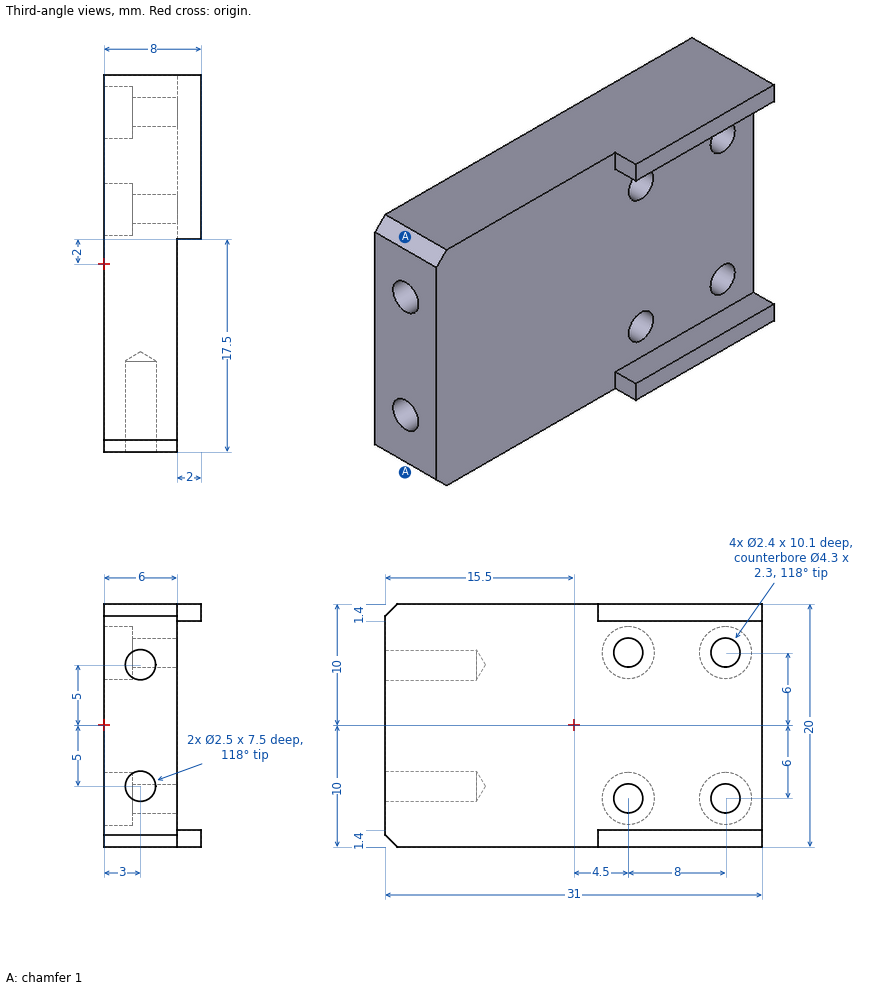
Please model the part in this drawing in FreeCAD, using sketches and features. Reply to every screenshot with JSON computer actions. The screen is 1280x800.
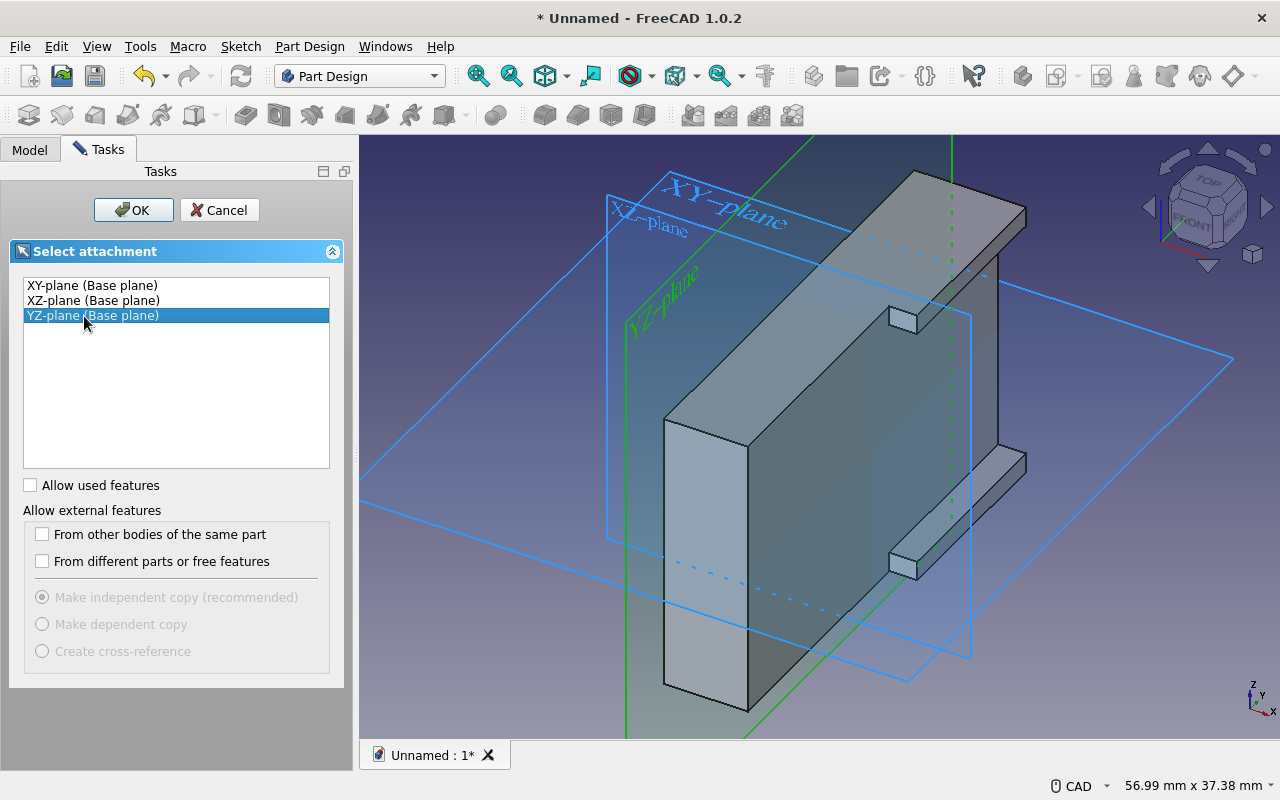
{"action": "left_click", "coordinate": [134, 210]}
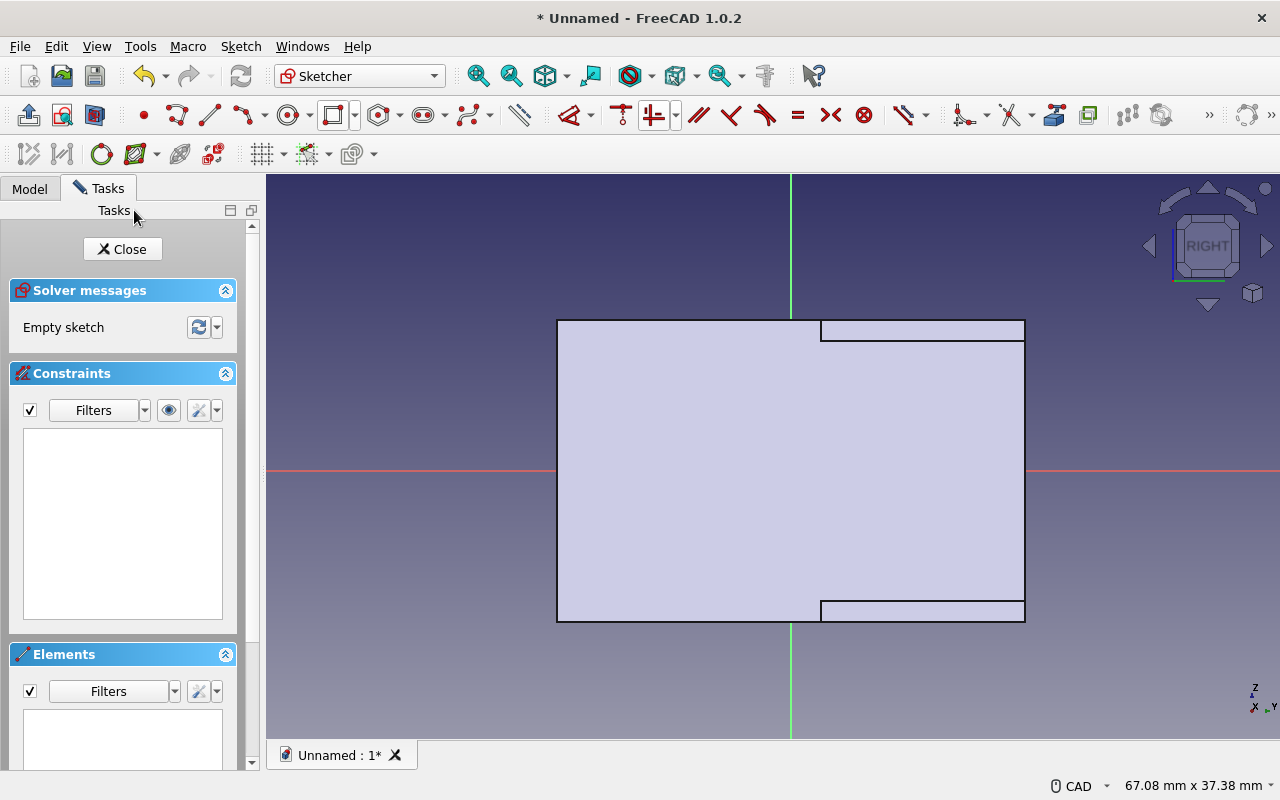
{"action": "left_click", "coordinate": [95, 116]}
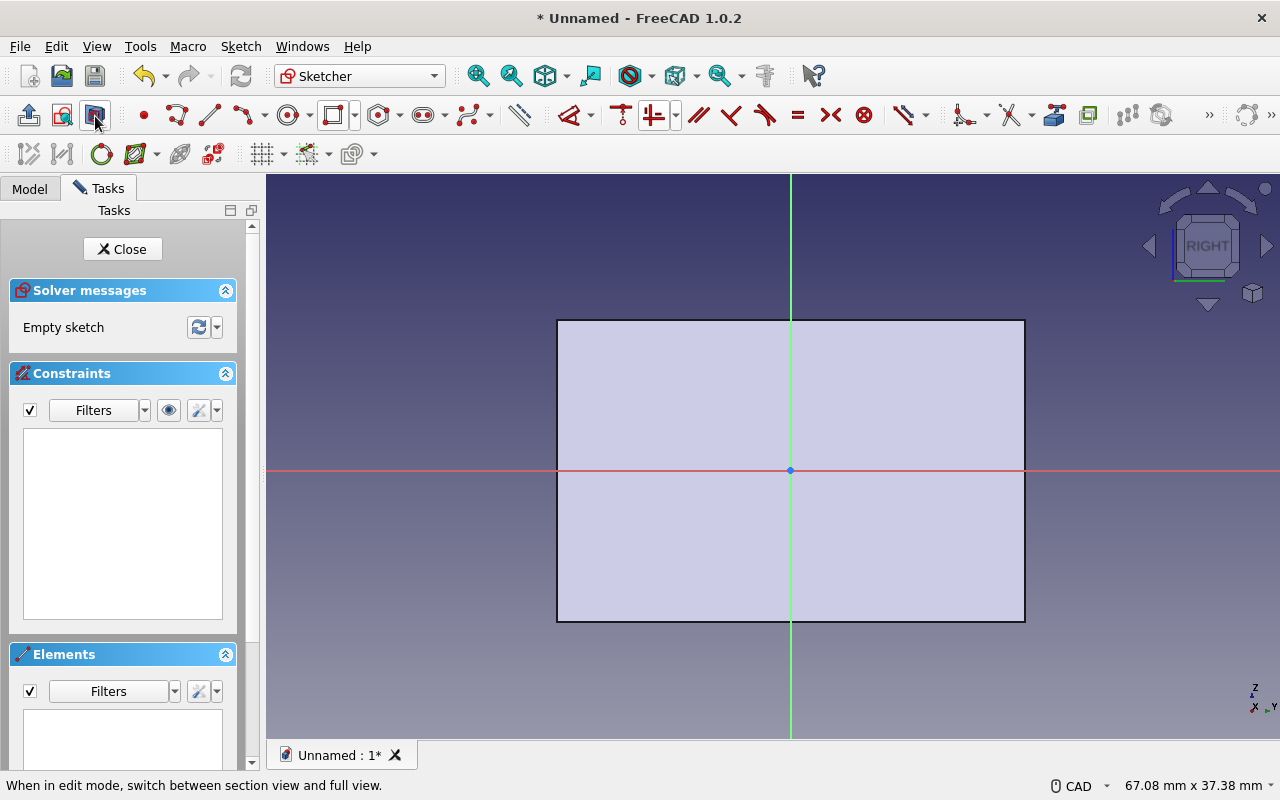
{"action": "scroll", "coordinate": [1115, 489], "scroll_direction": "up", "scroll_amount": 3}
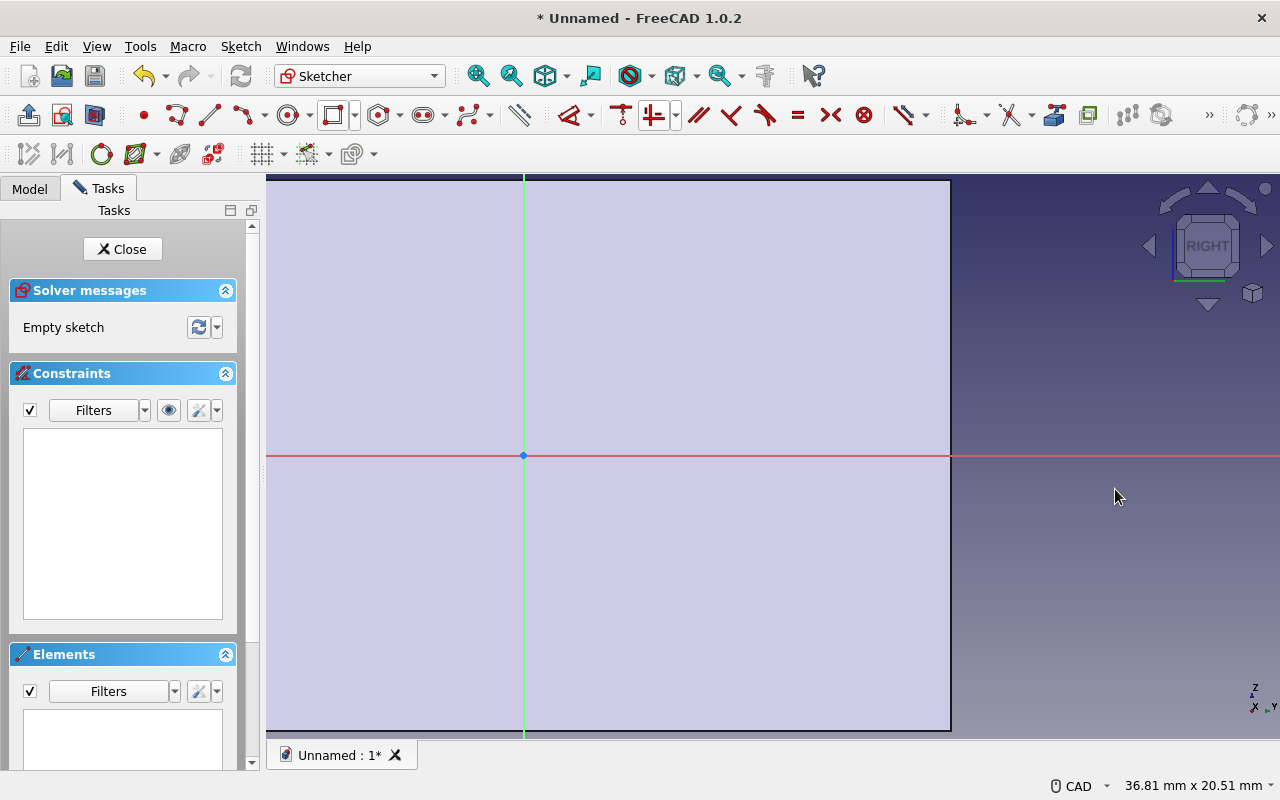
{"action": "left_click", "coordinate": [288, 116]}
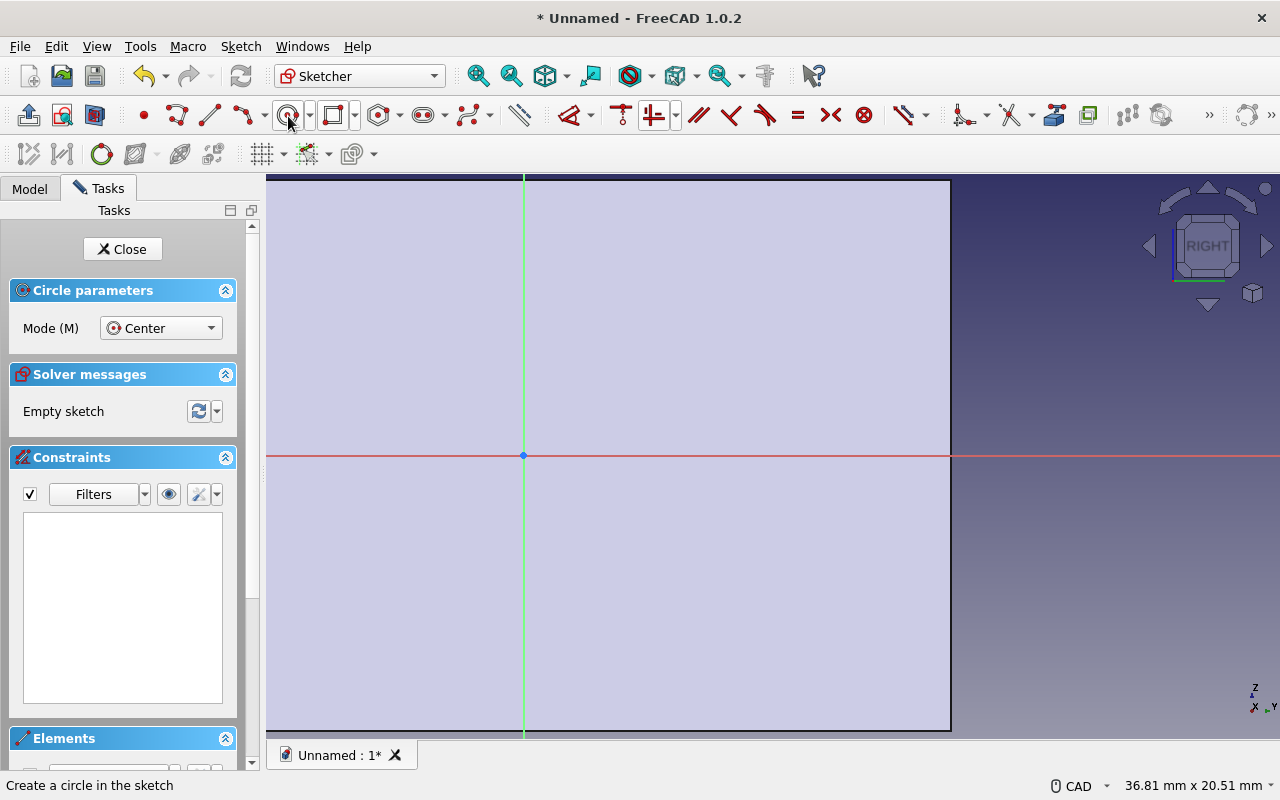
{"action": "left_click", "coordinate": [868, 290]}
{"action": "left_click", "coordinate": [891, 267]}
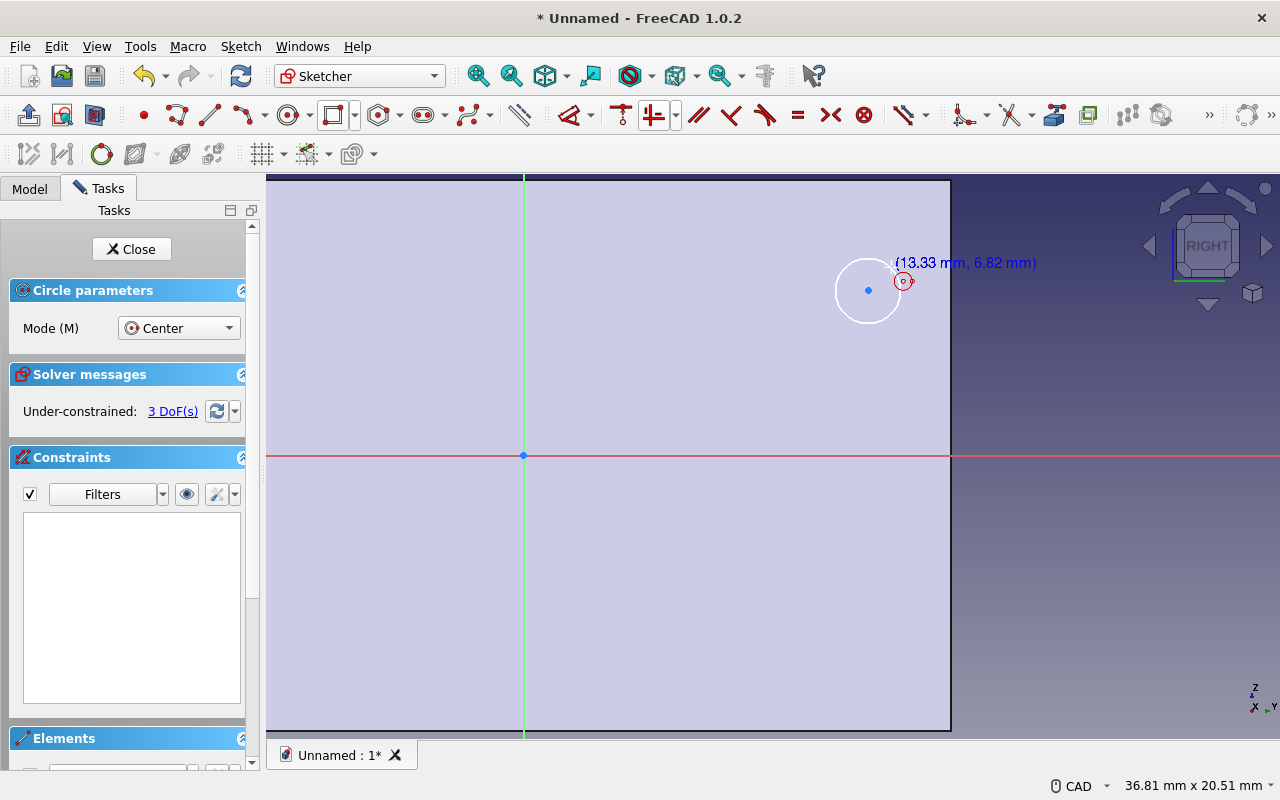
{"action": "left_click", "coordinate": [868, 621]}
{"action": "left_click", "coordinate": [891, 598]}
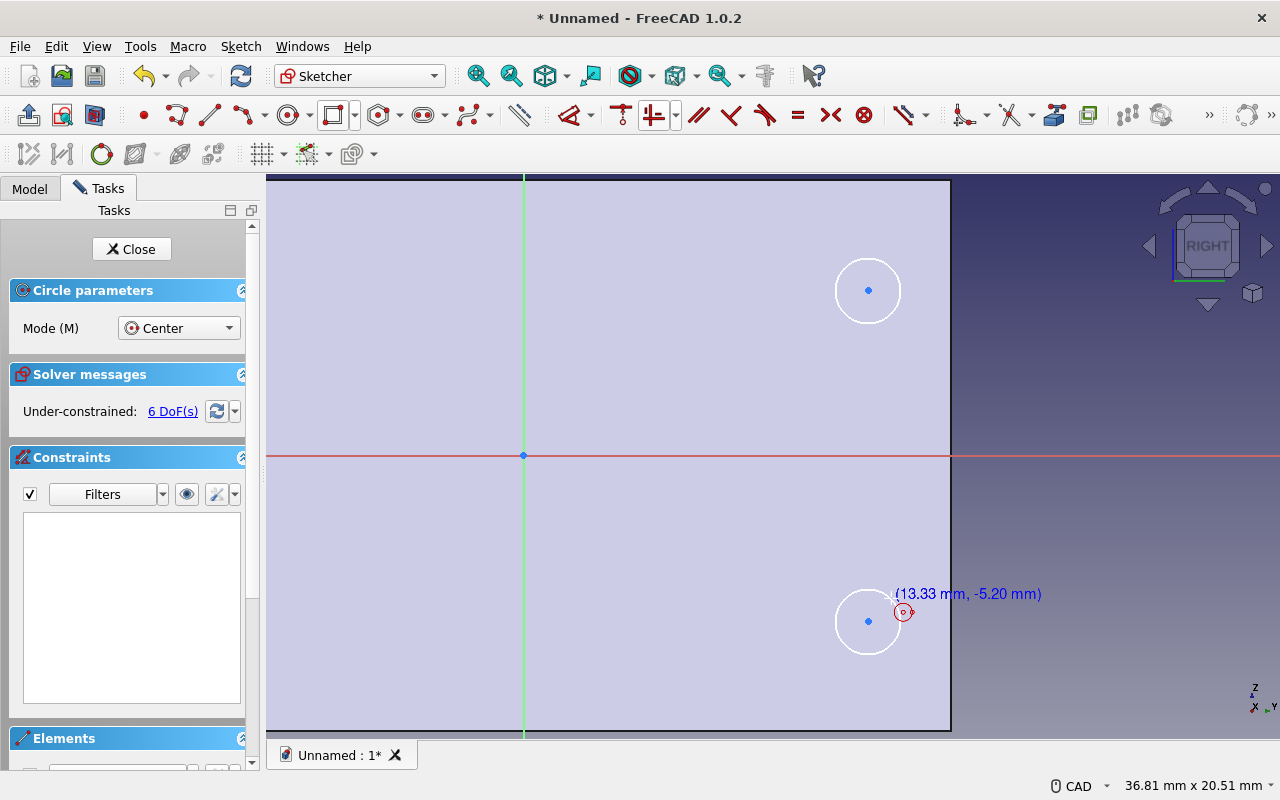
{"action": "left_click", "coordinate": [648, 621]}
{"action": "left_click", "coordinate": [671, 598]}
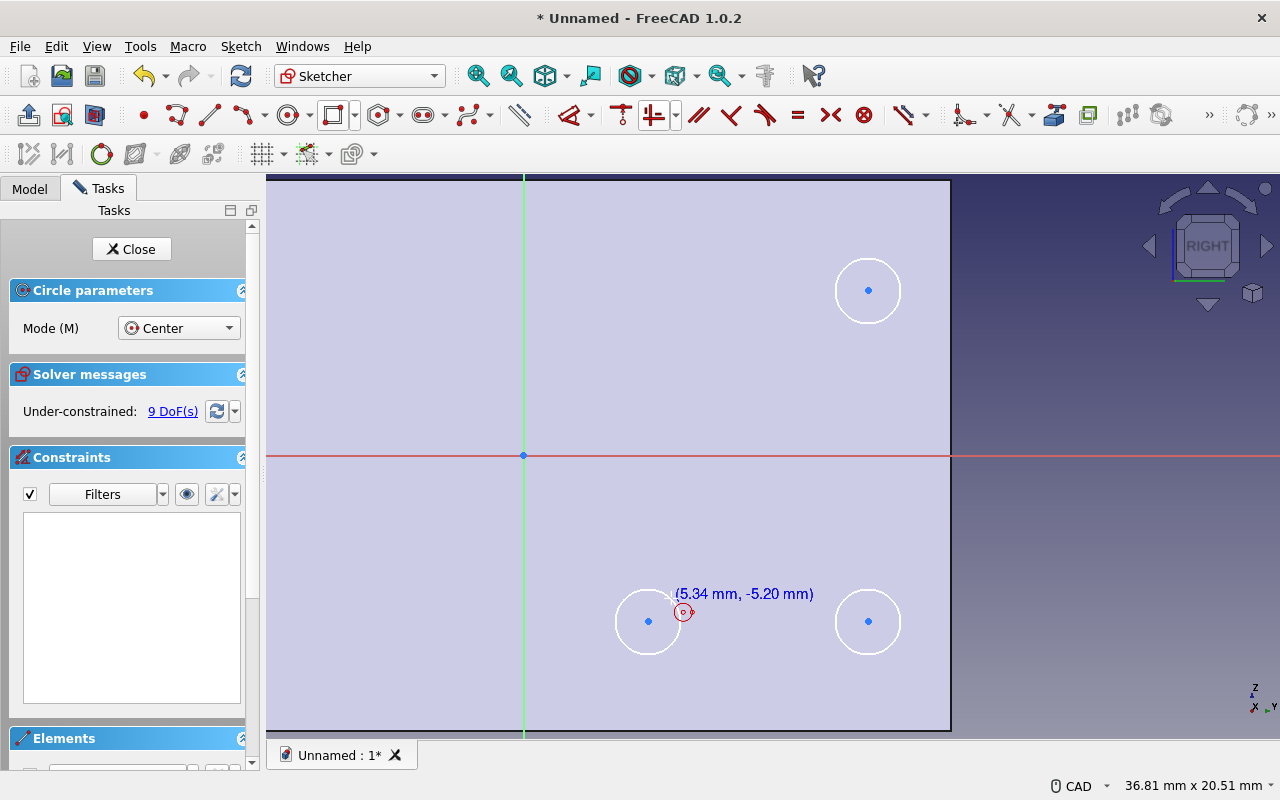
{"action": "left_click", "coordinate": [648, 290]}
{"action": "left_click", "coordinate": [671, 267]}
{"action": "key", "text": "Escape"}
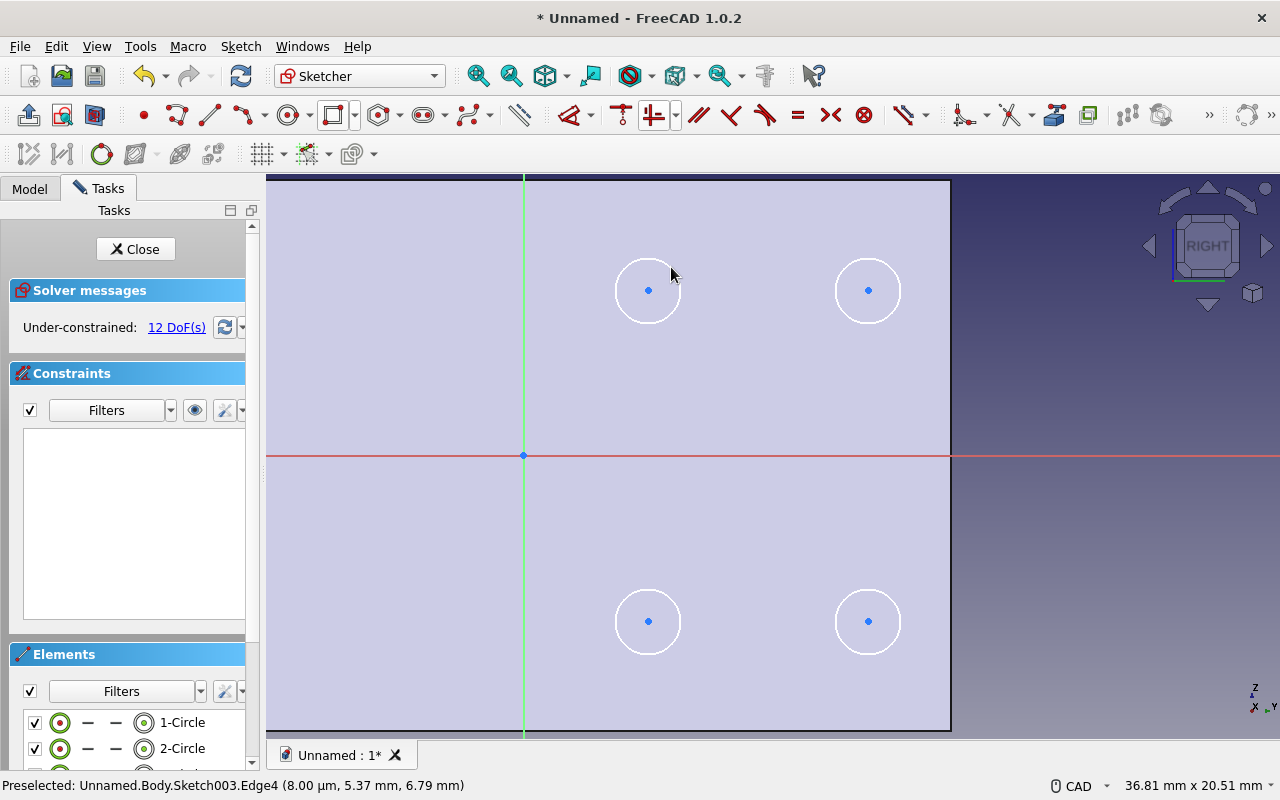
{"action": "left_click", "coordinate": [891, 268]}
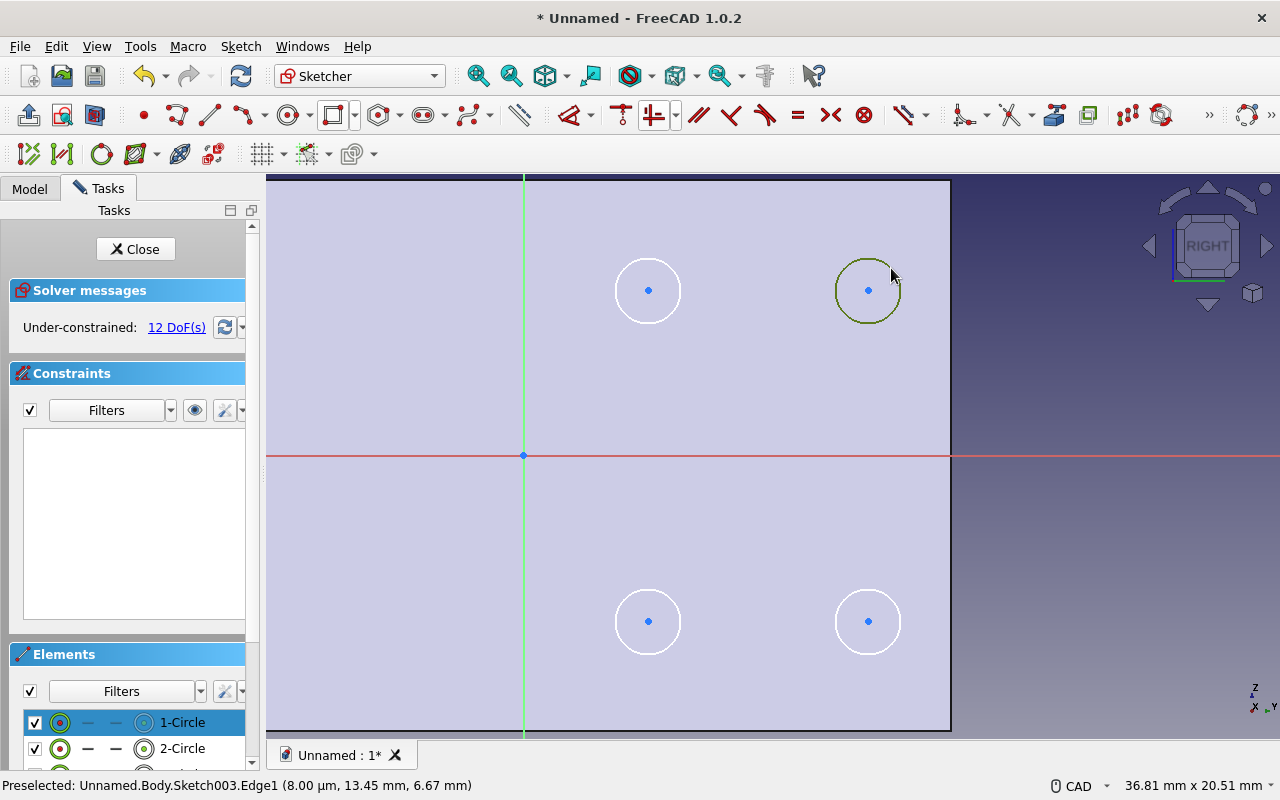
{"action": "left_click", "coordinate": [891, 599]}